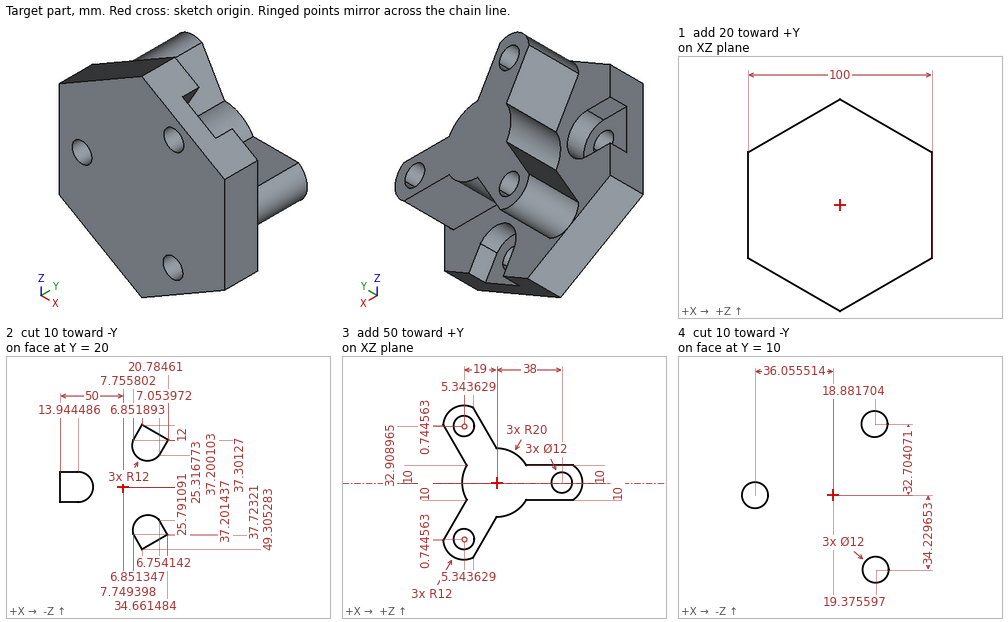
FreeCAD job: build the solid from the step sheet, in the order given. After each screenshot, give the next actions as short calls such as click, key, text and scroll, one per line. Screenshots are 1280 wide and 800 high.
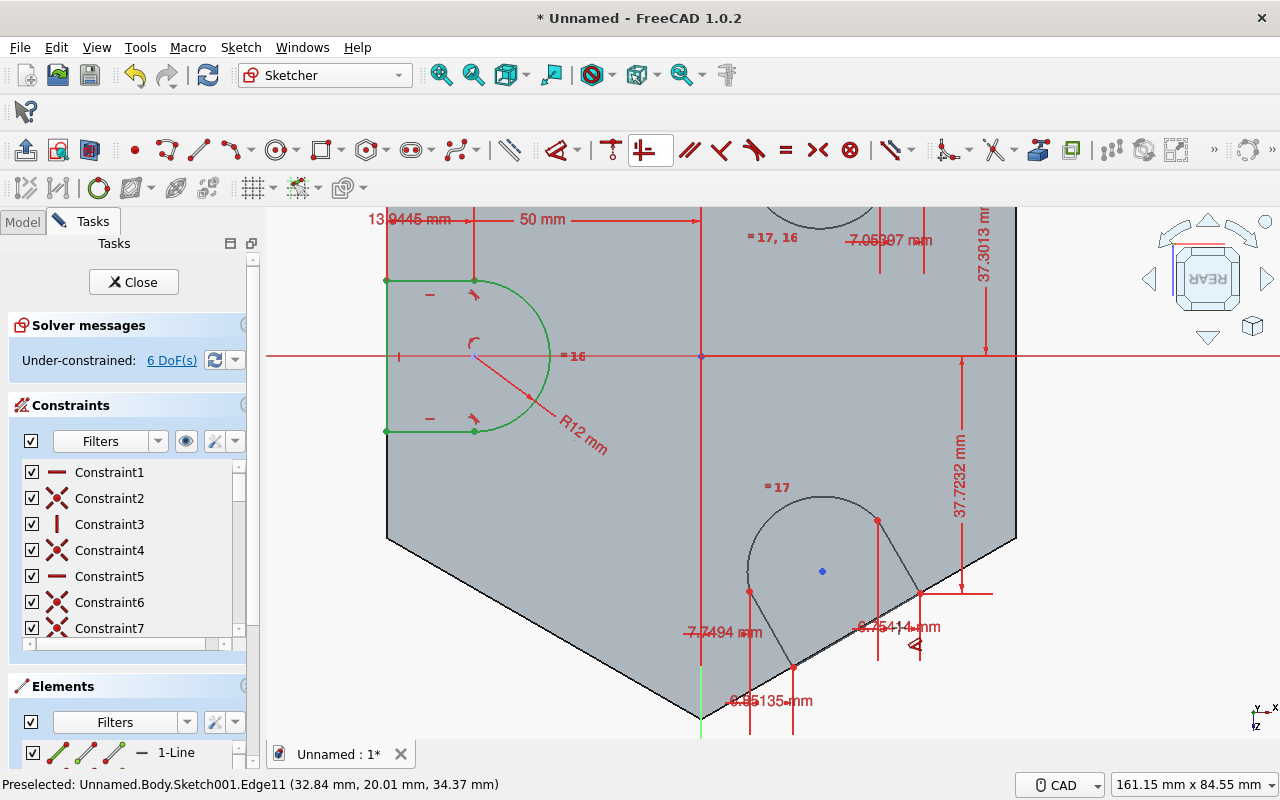
scroll(764, 615, down, 3)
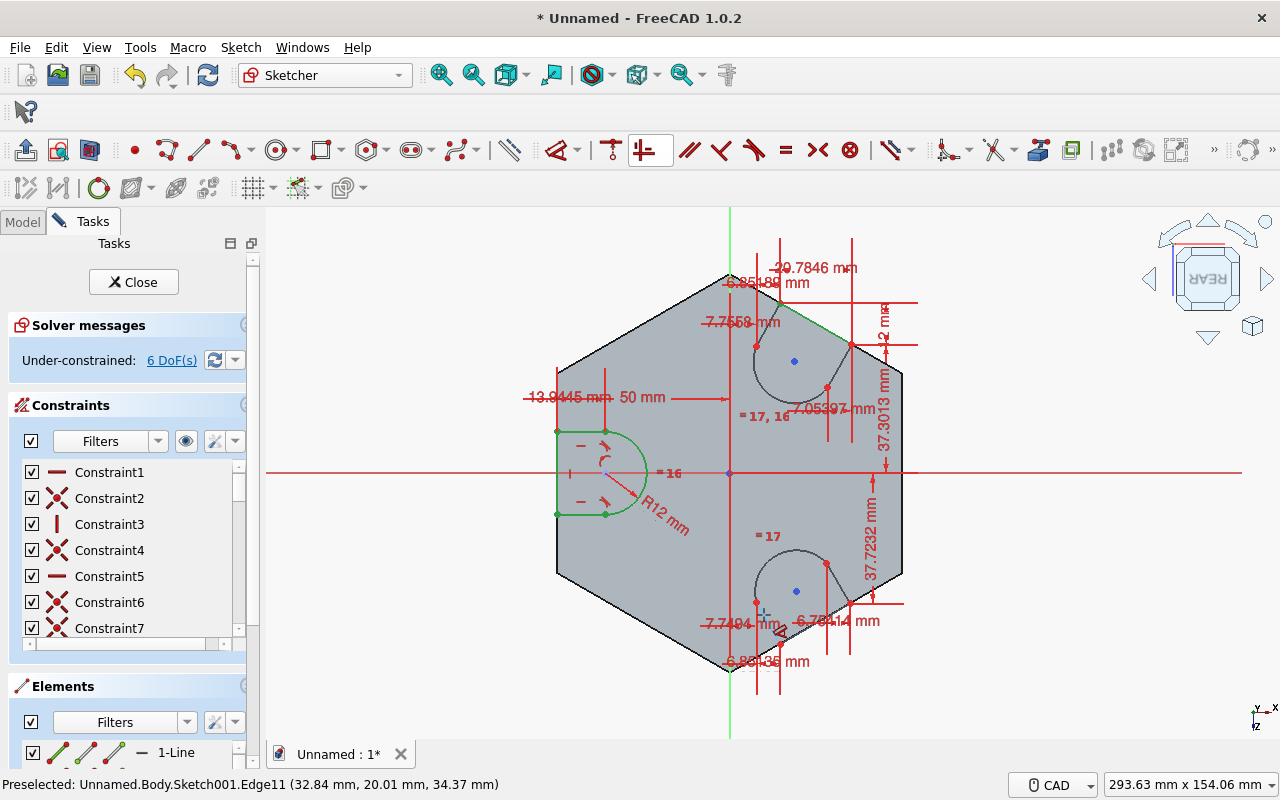
click(828, 387)
click(862, 430)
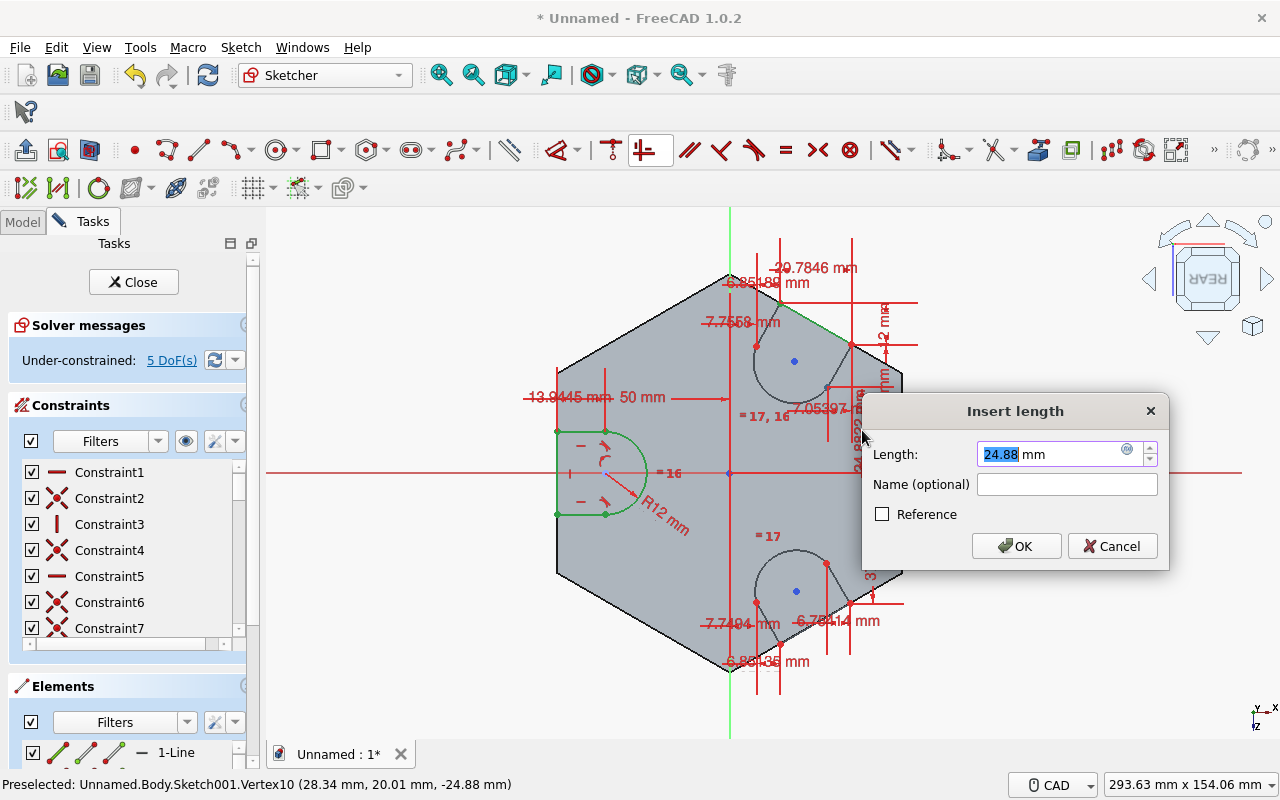
text(25.316773)
key(Return)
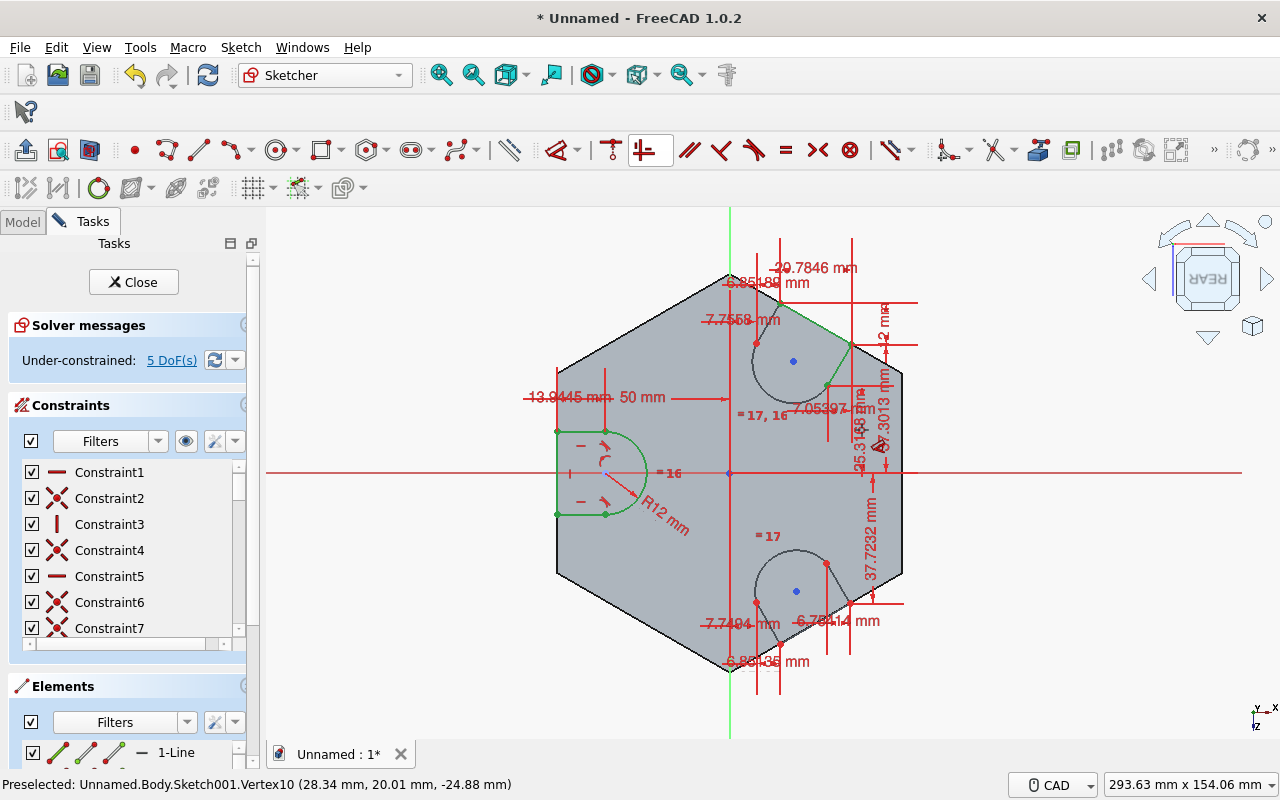
click(757, 344)
click(791, 379)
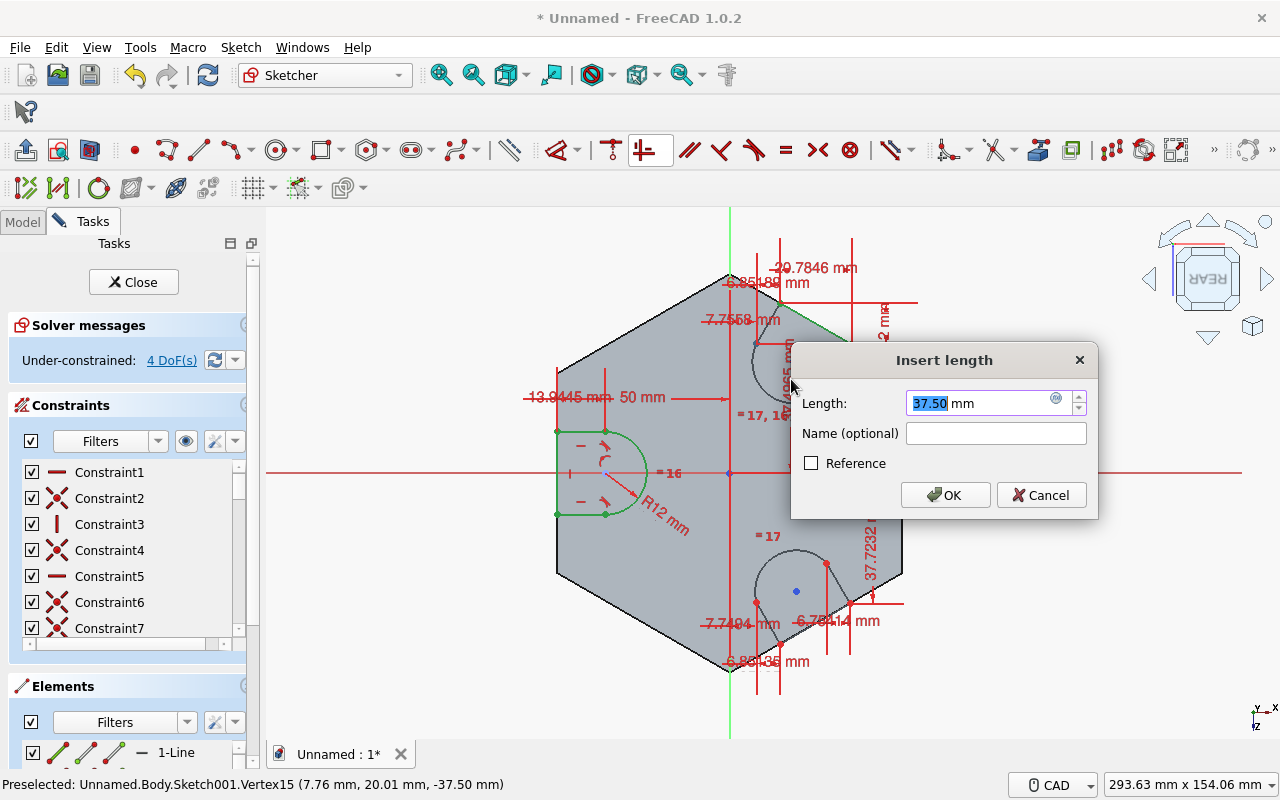
text(37.200103)
key(Return)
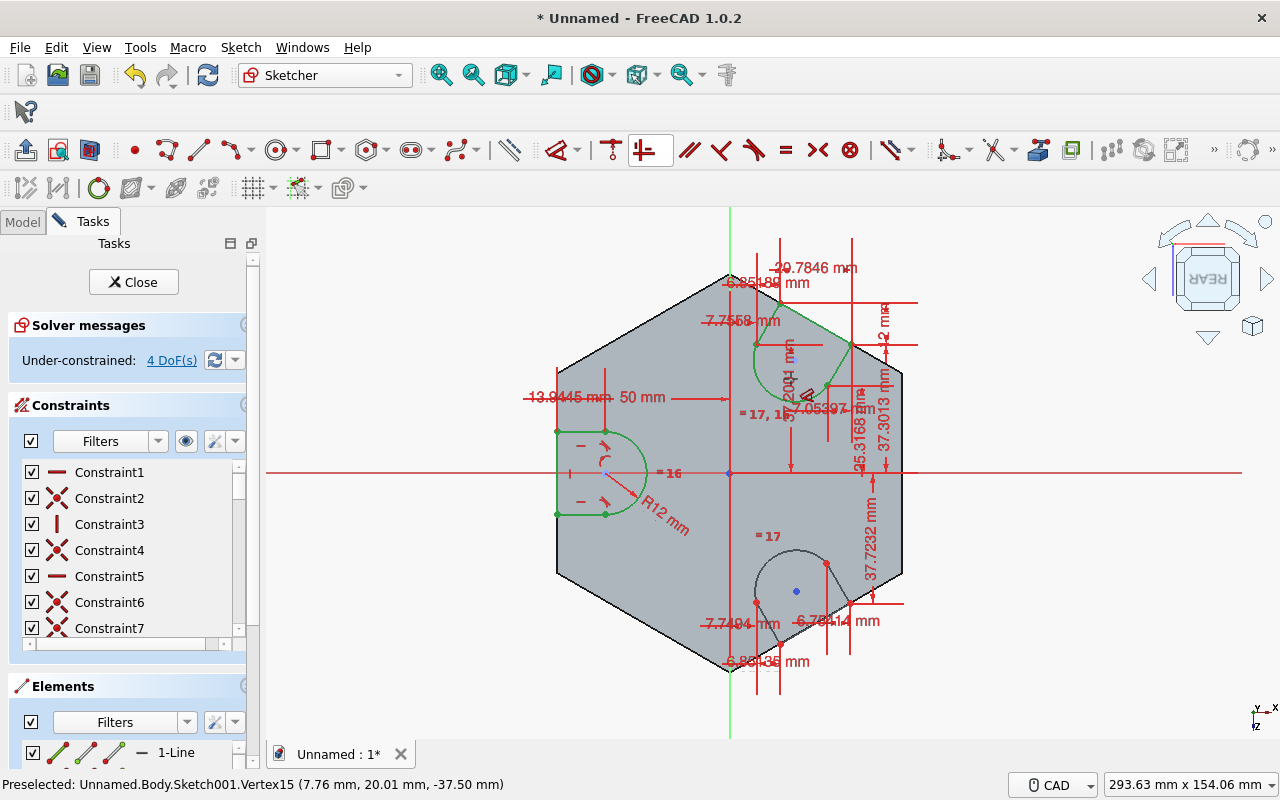
click(757, 602)
click(791, 508)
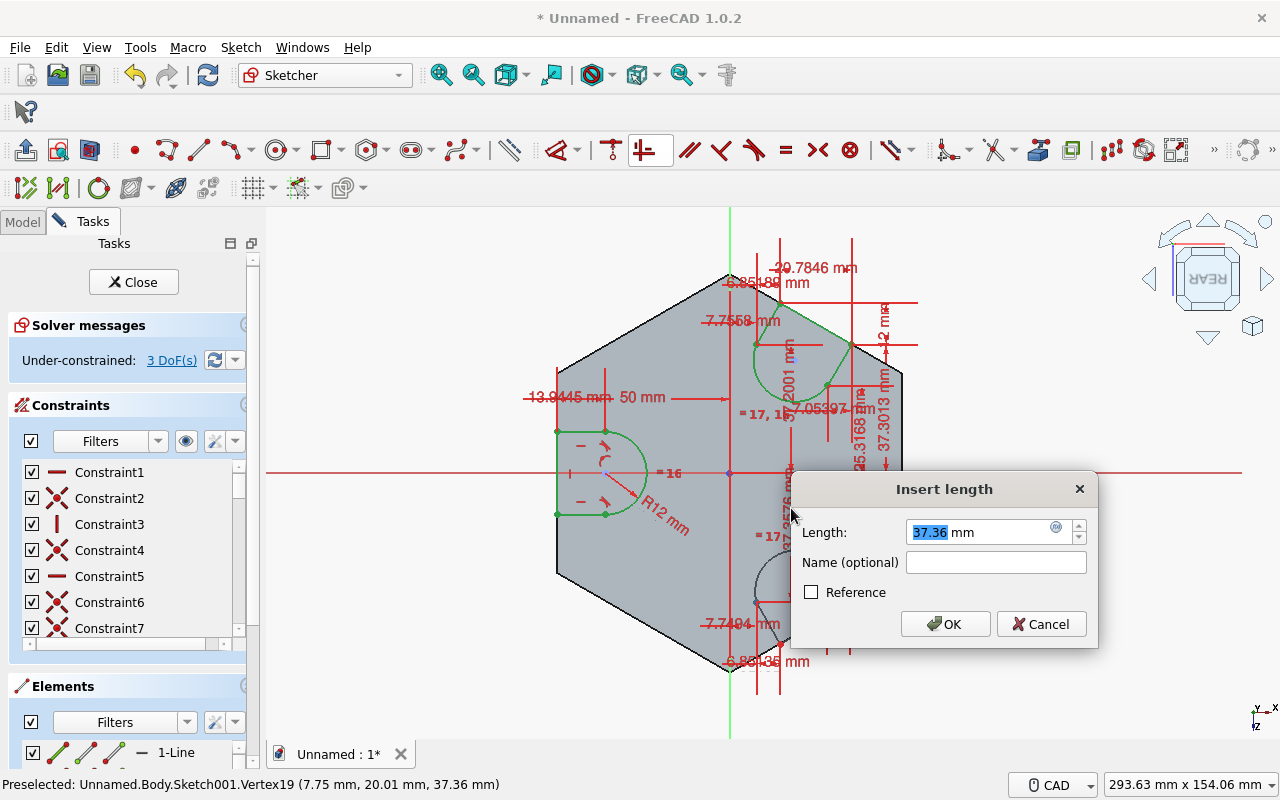
text(37.201437)
key(Return)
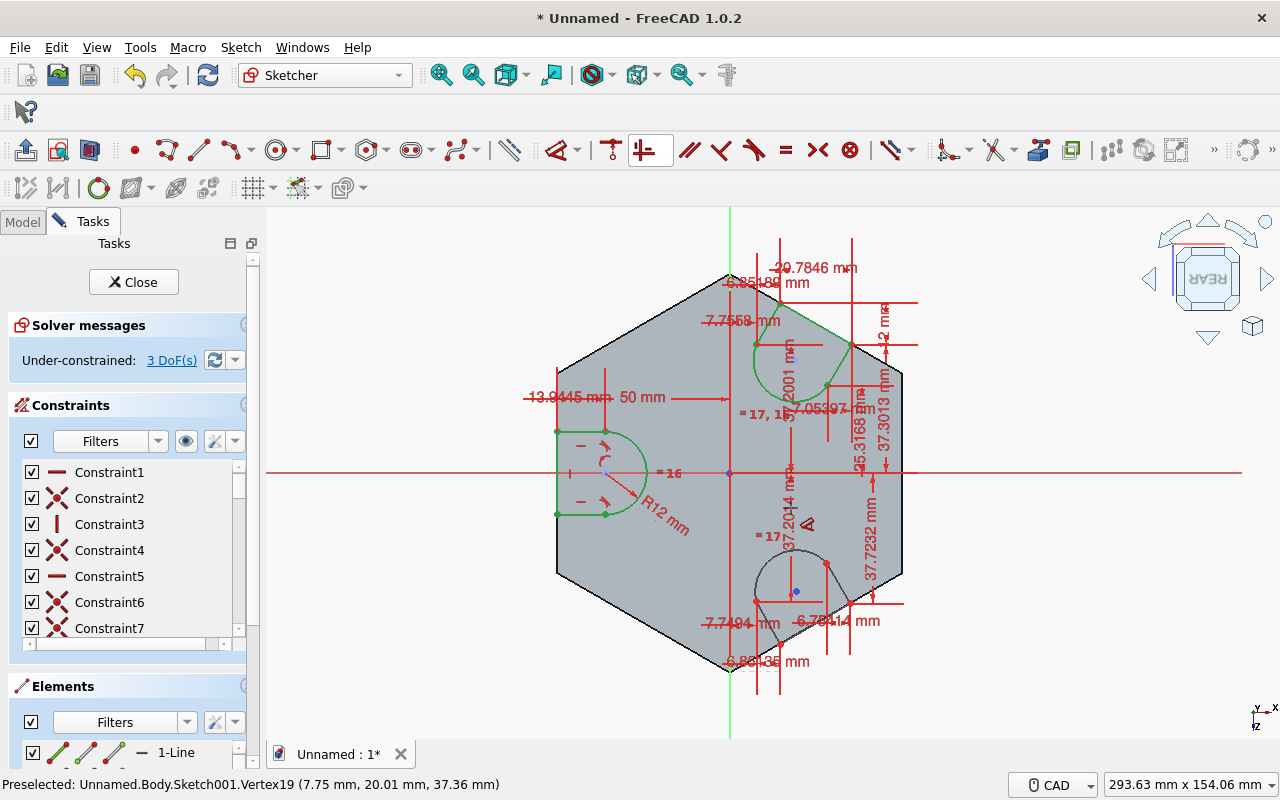
click(780, 644)
click(814, 598)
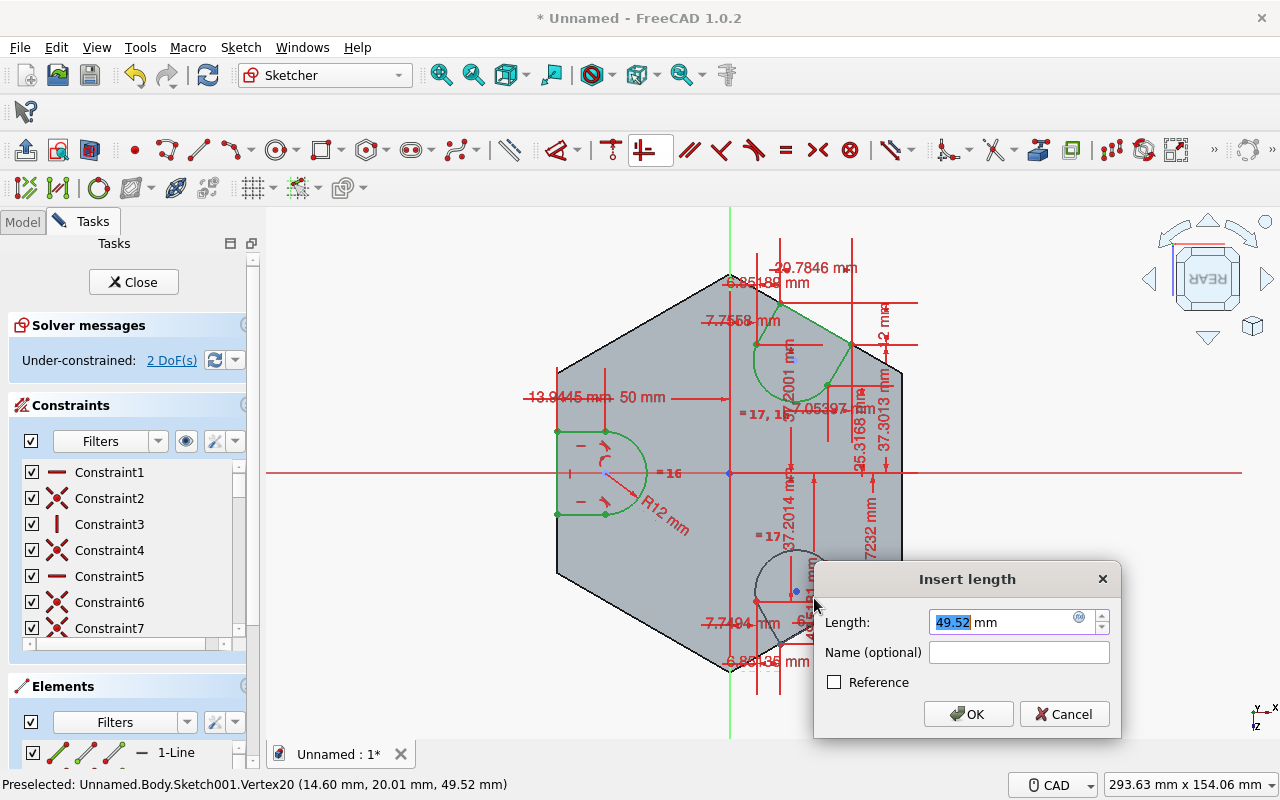
text(49.305283)
key(Return)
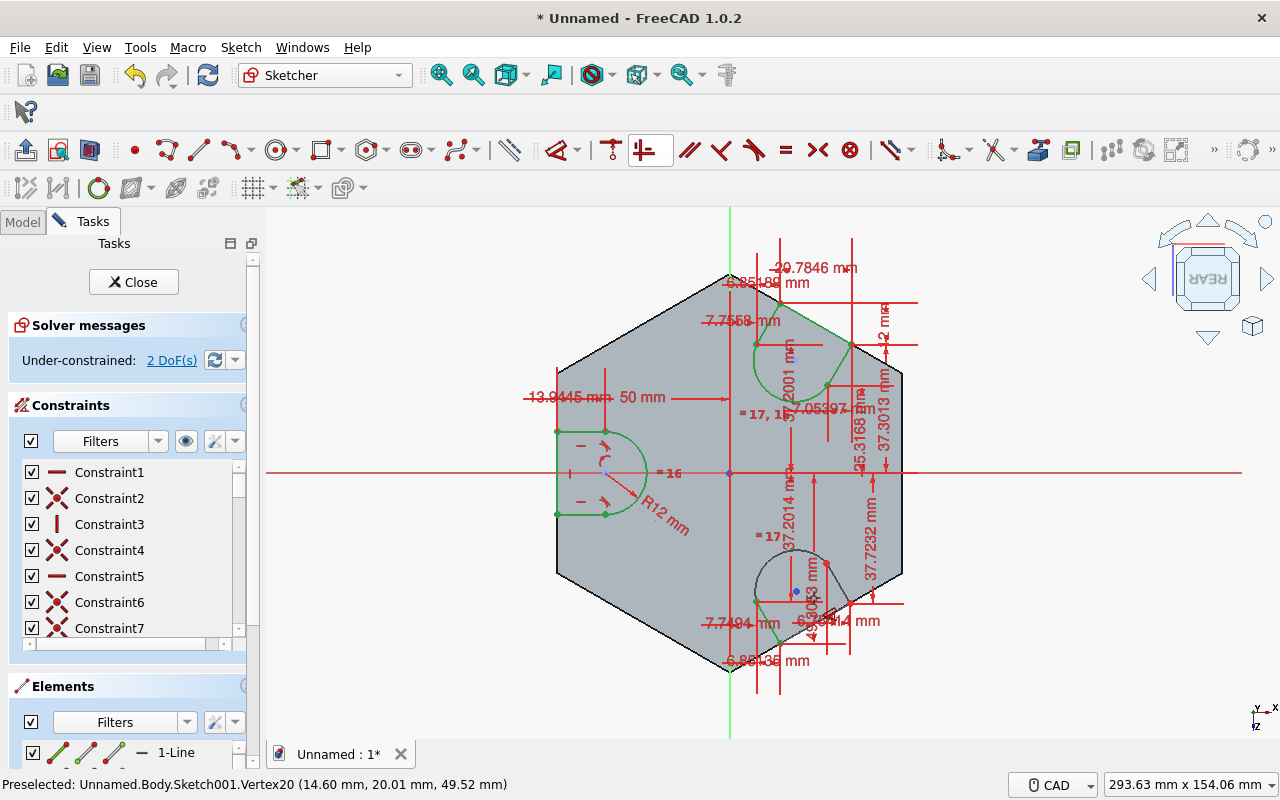
click(850, 604)
click(790, 439)